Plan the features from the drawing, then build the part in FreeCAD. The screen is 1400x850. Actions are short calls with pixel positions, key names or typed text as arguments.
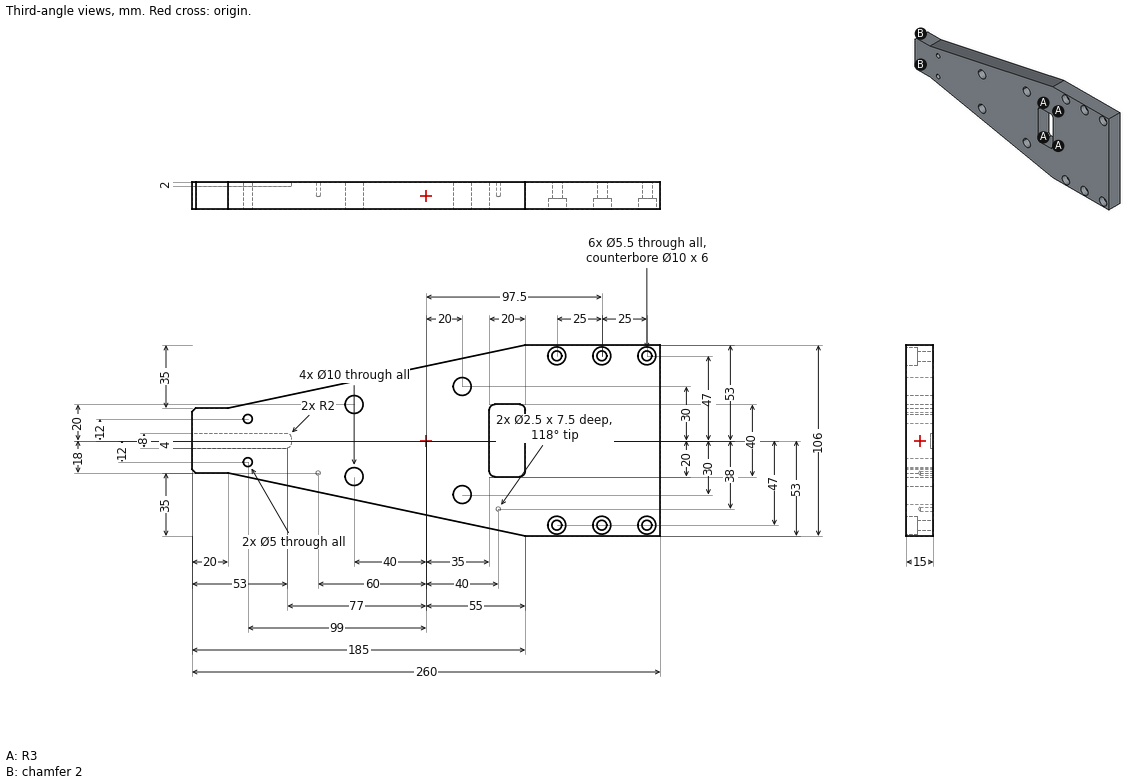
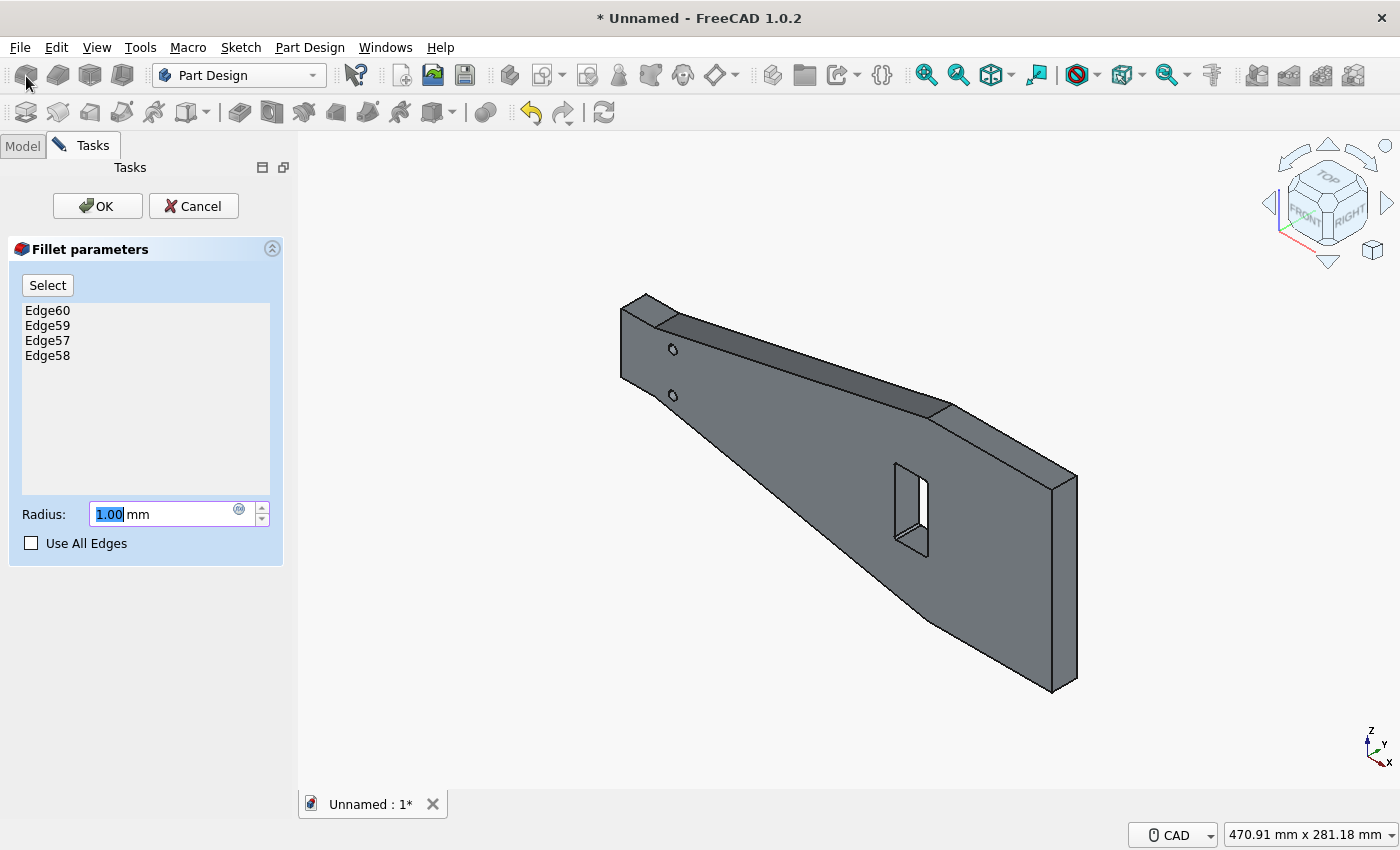
text(3)
key(Tab)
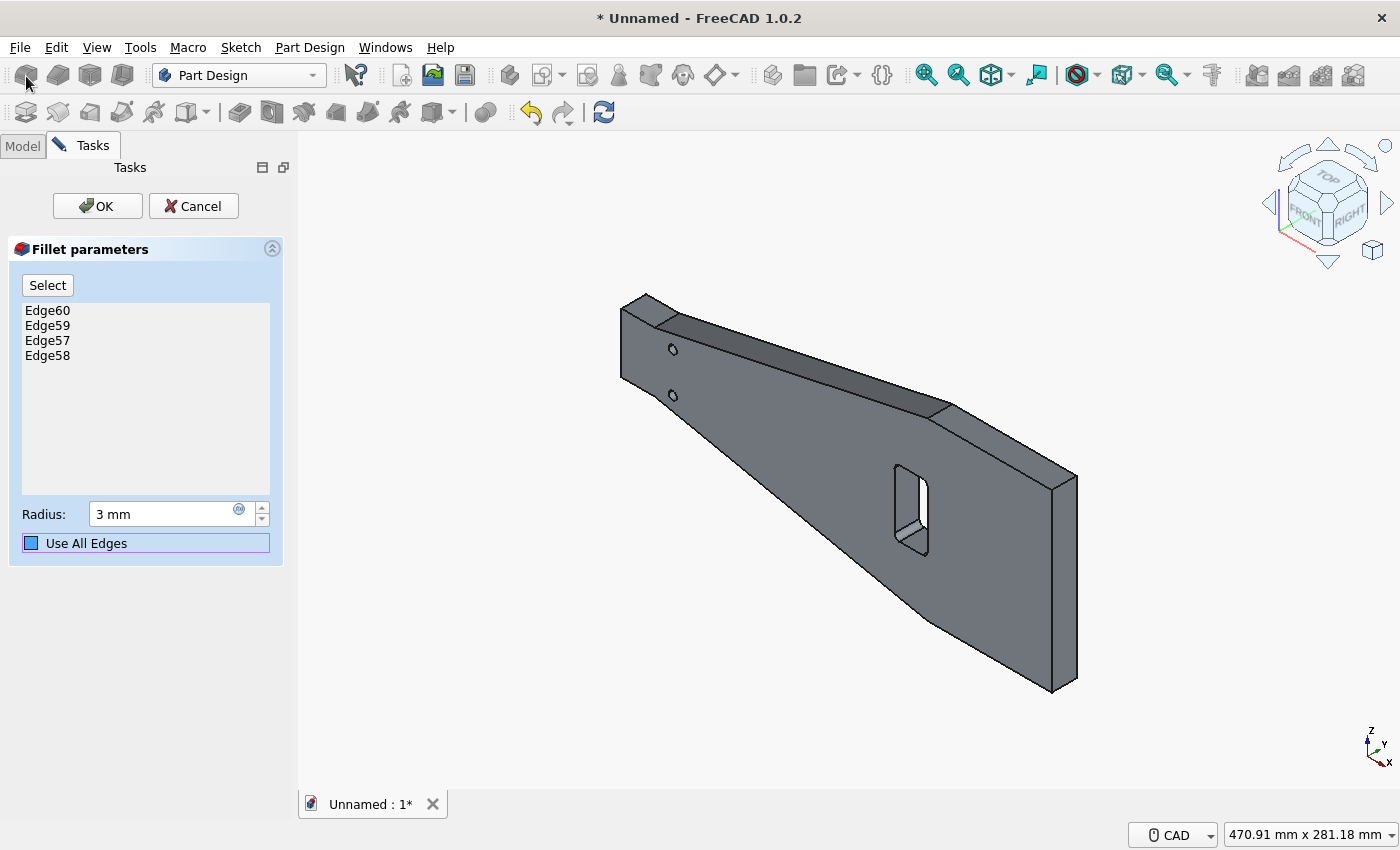
click(98, 206)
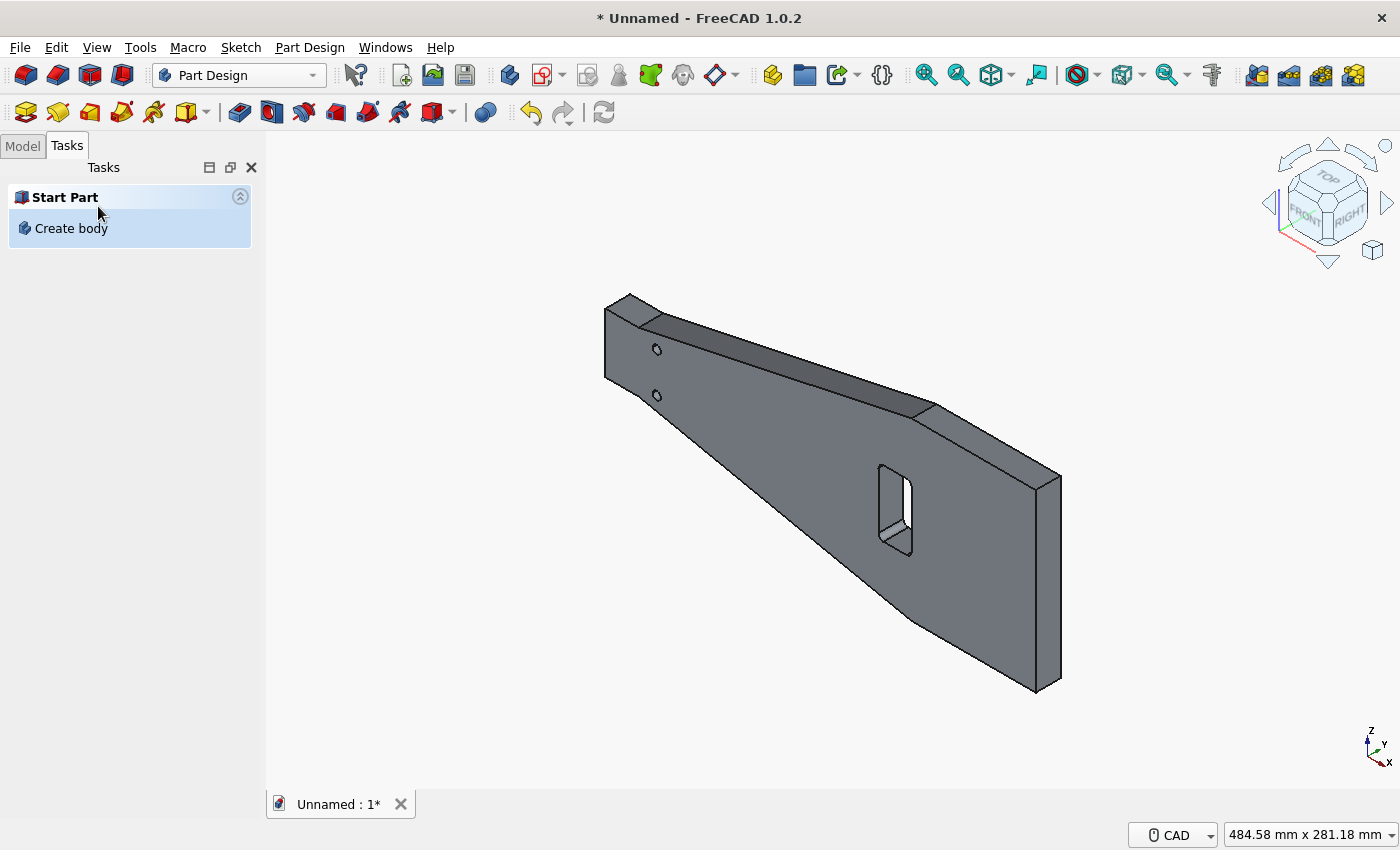
click(821, 466)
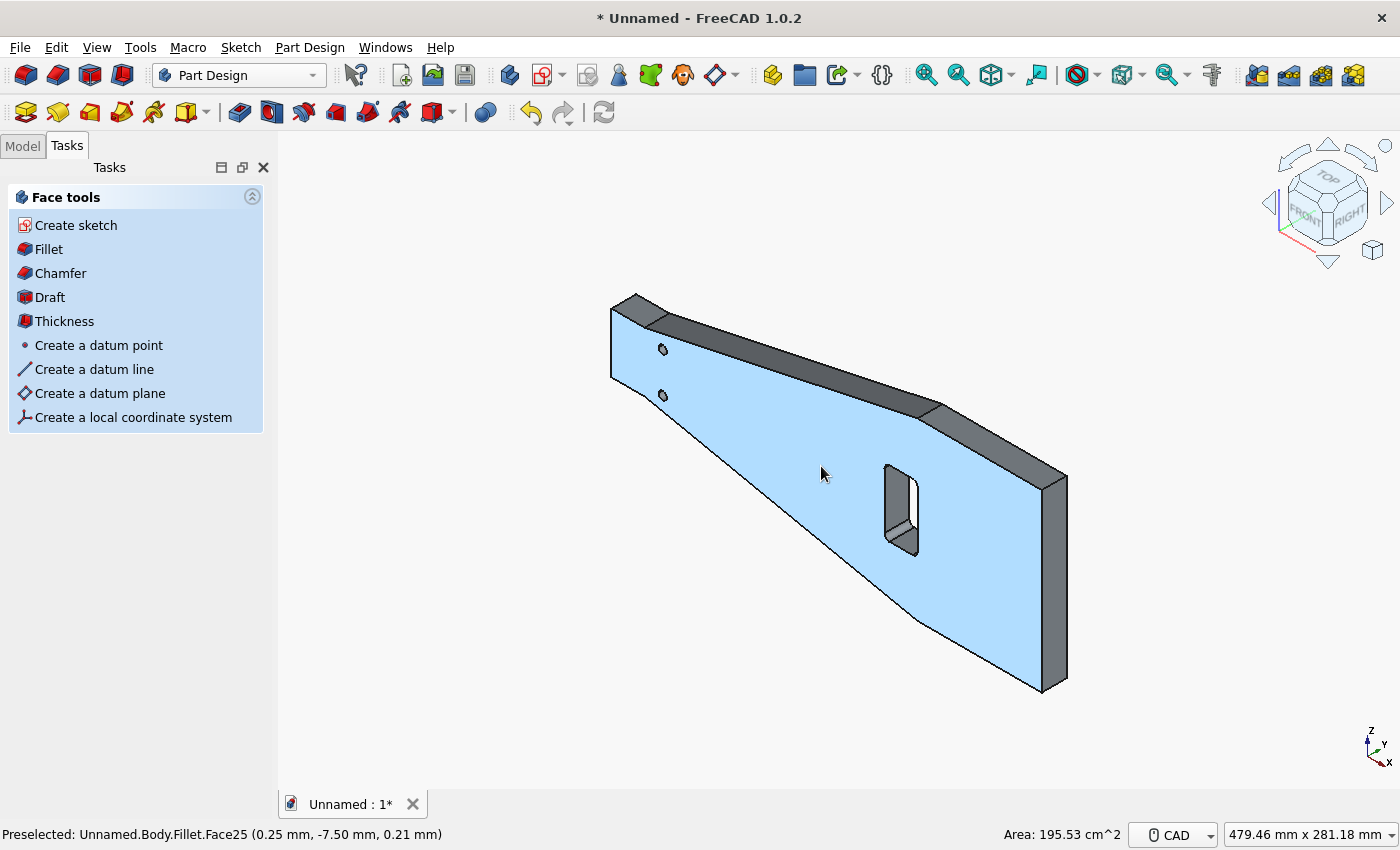
click(542, 76)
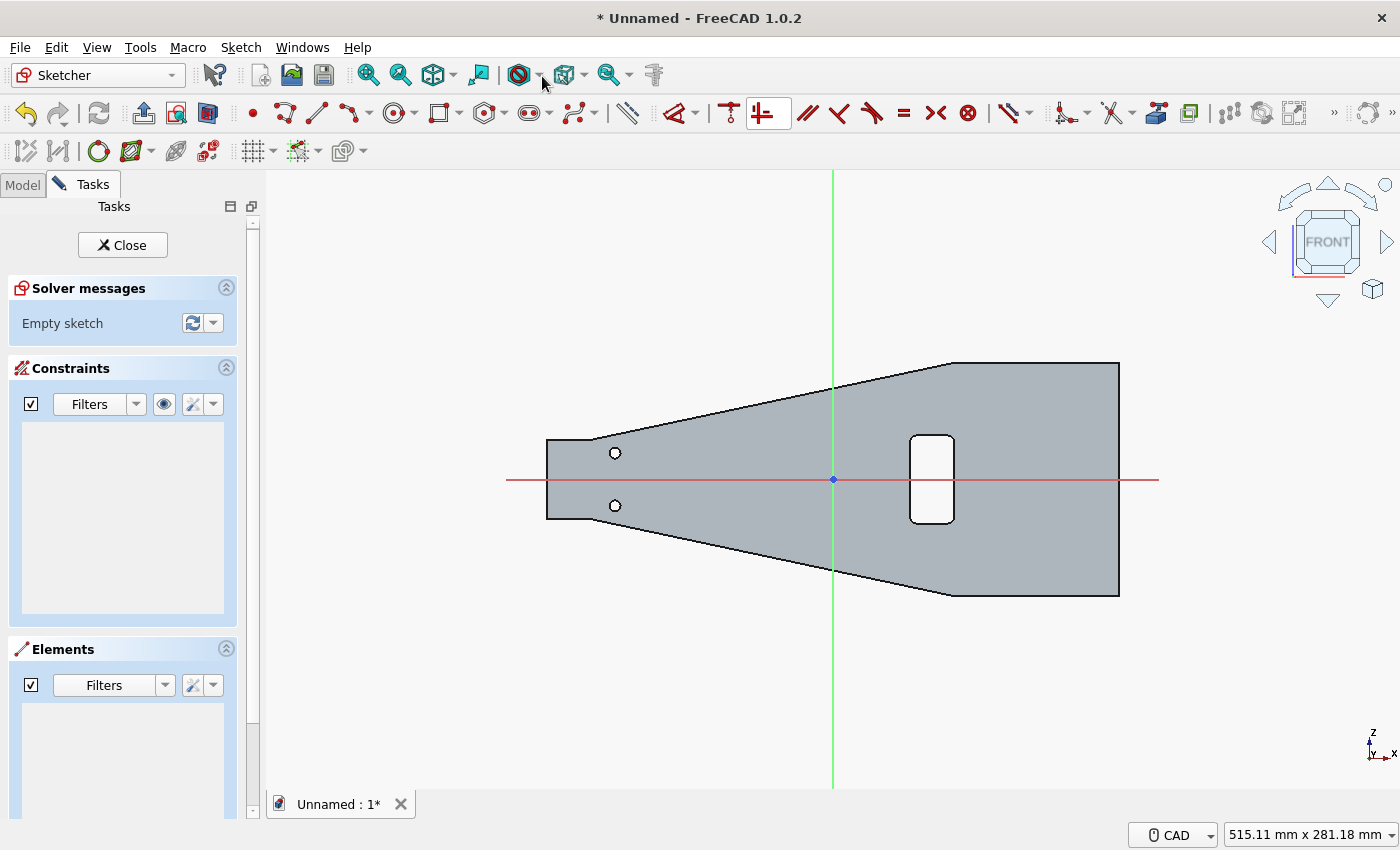
scroll(1222, 480, up, 3)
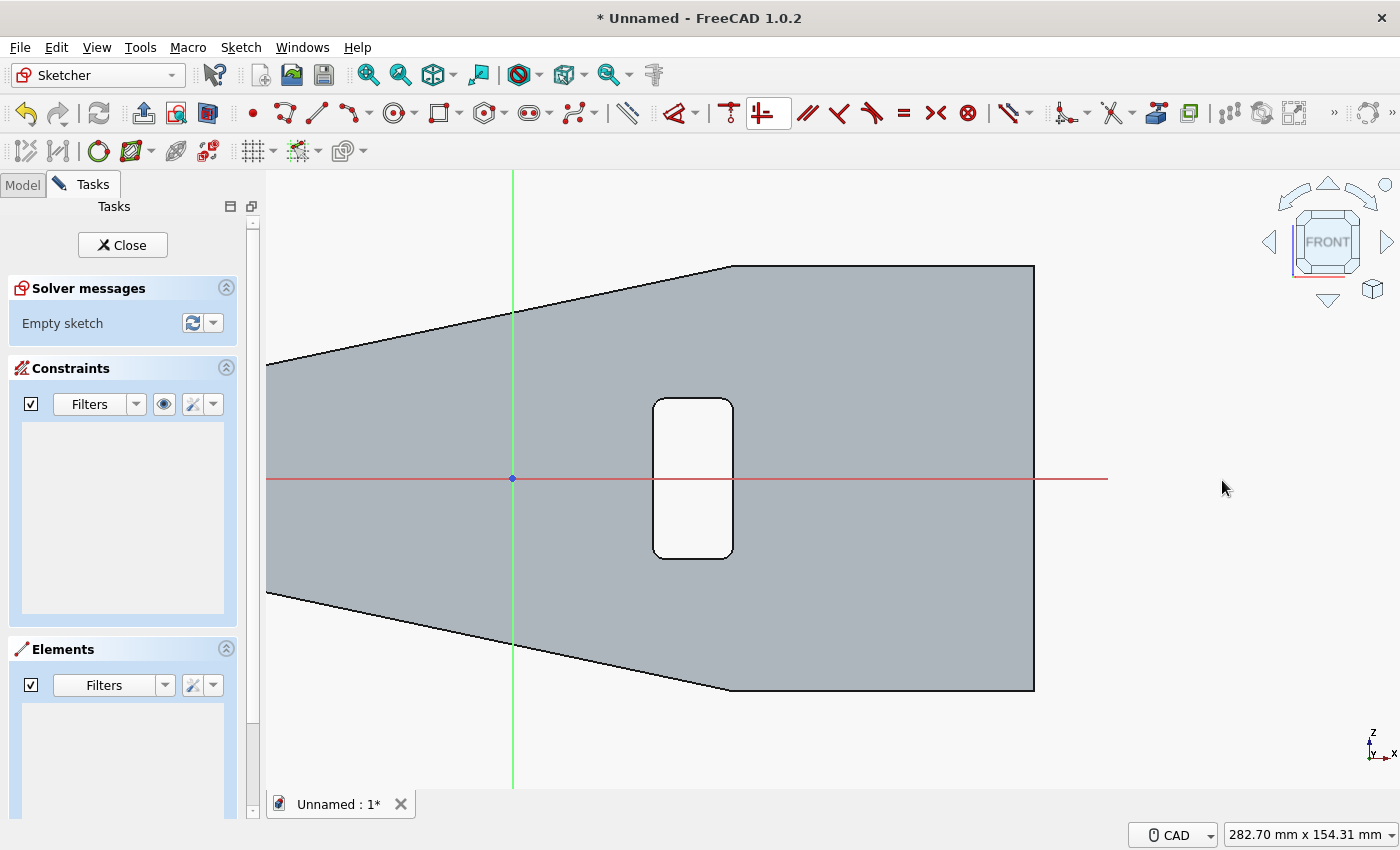
key(g)
key(c)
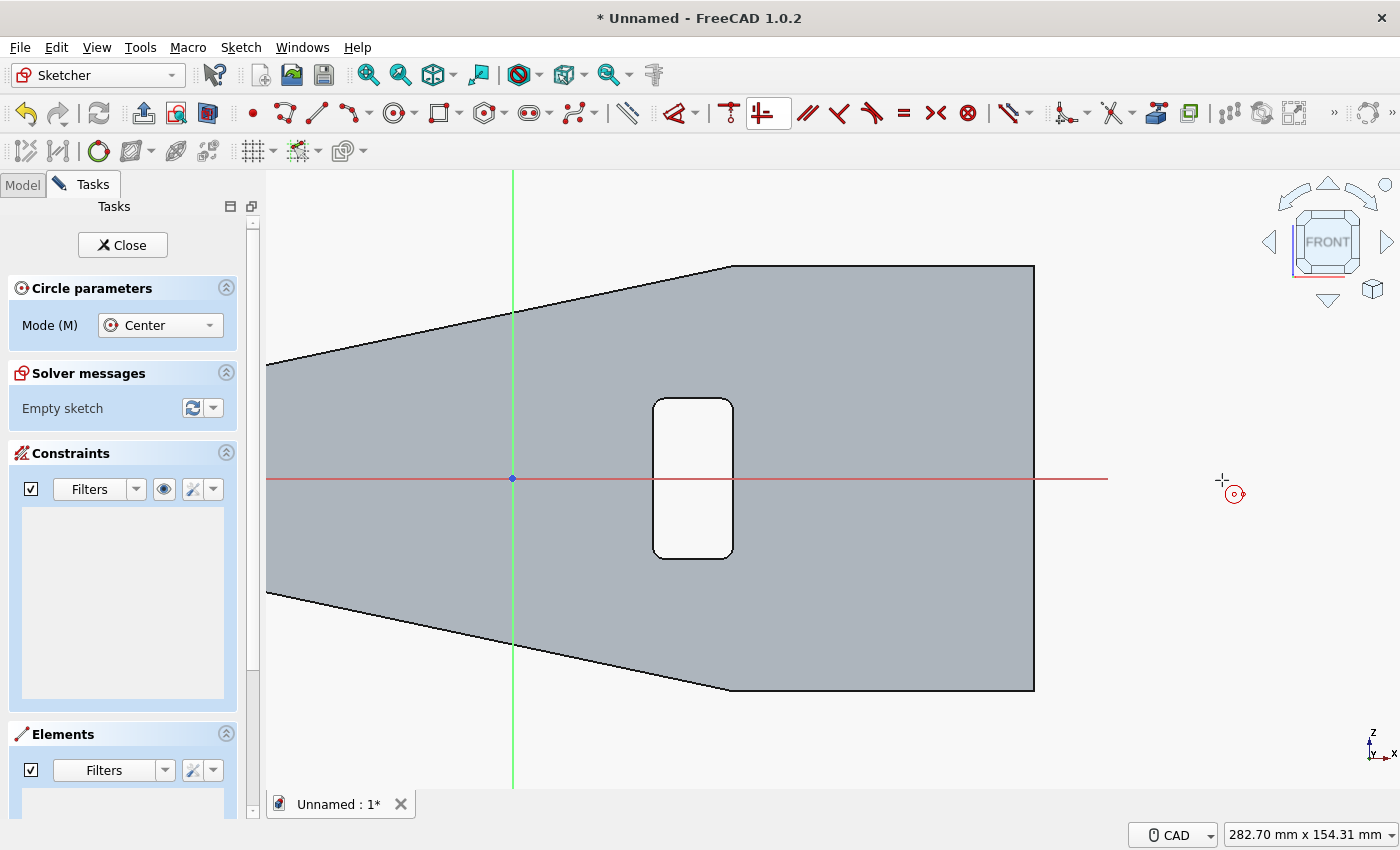
scroll(1004, 290, up, 4)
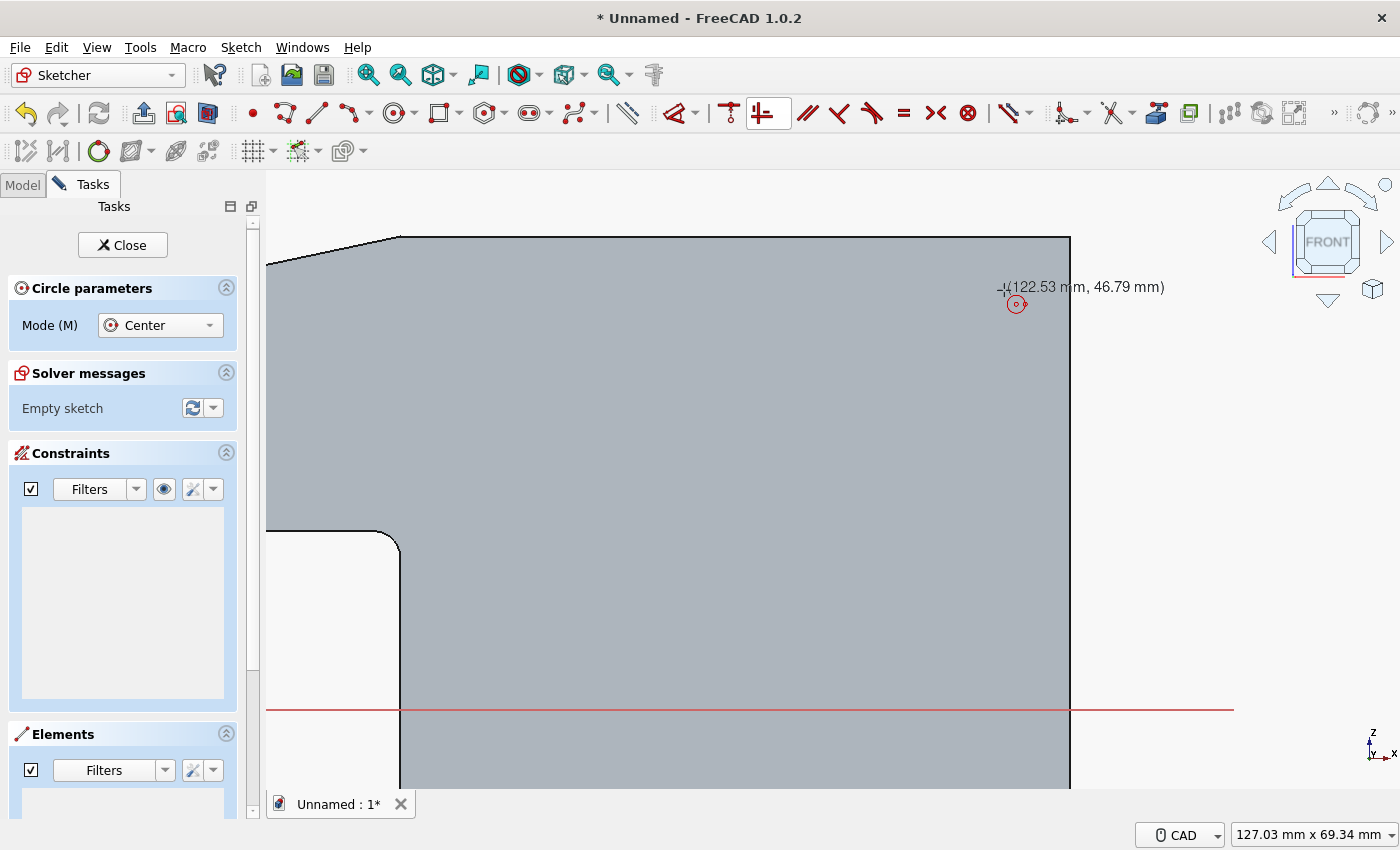
click(1003, 290)
click(1020, 273)